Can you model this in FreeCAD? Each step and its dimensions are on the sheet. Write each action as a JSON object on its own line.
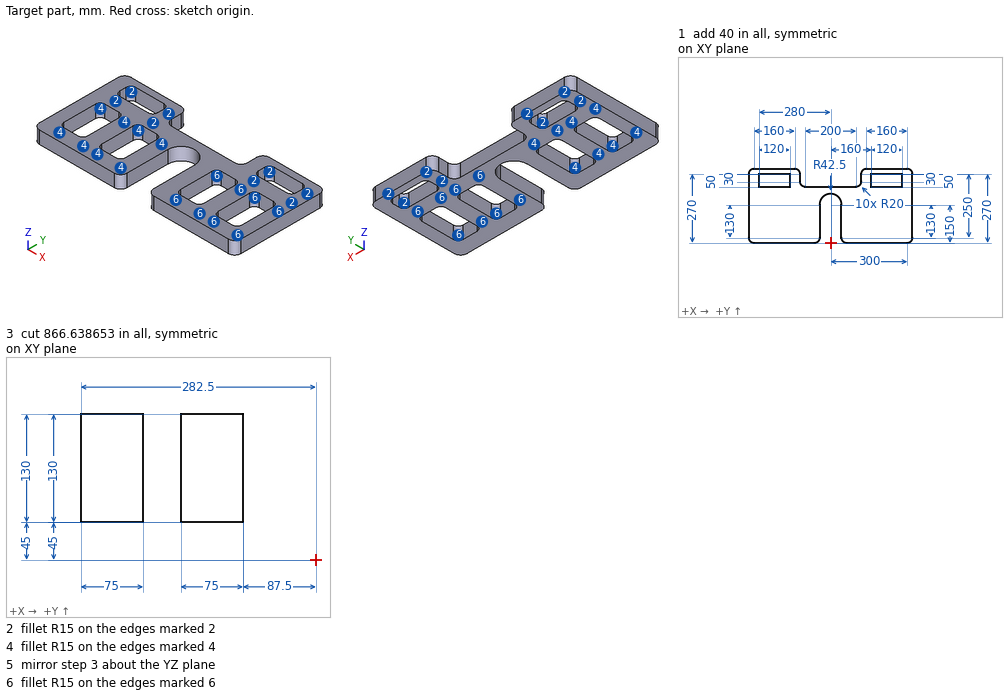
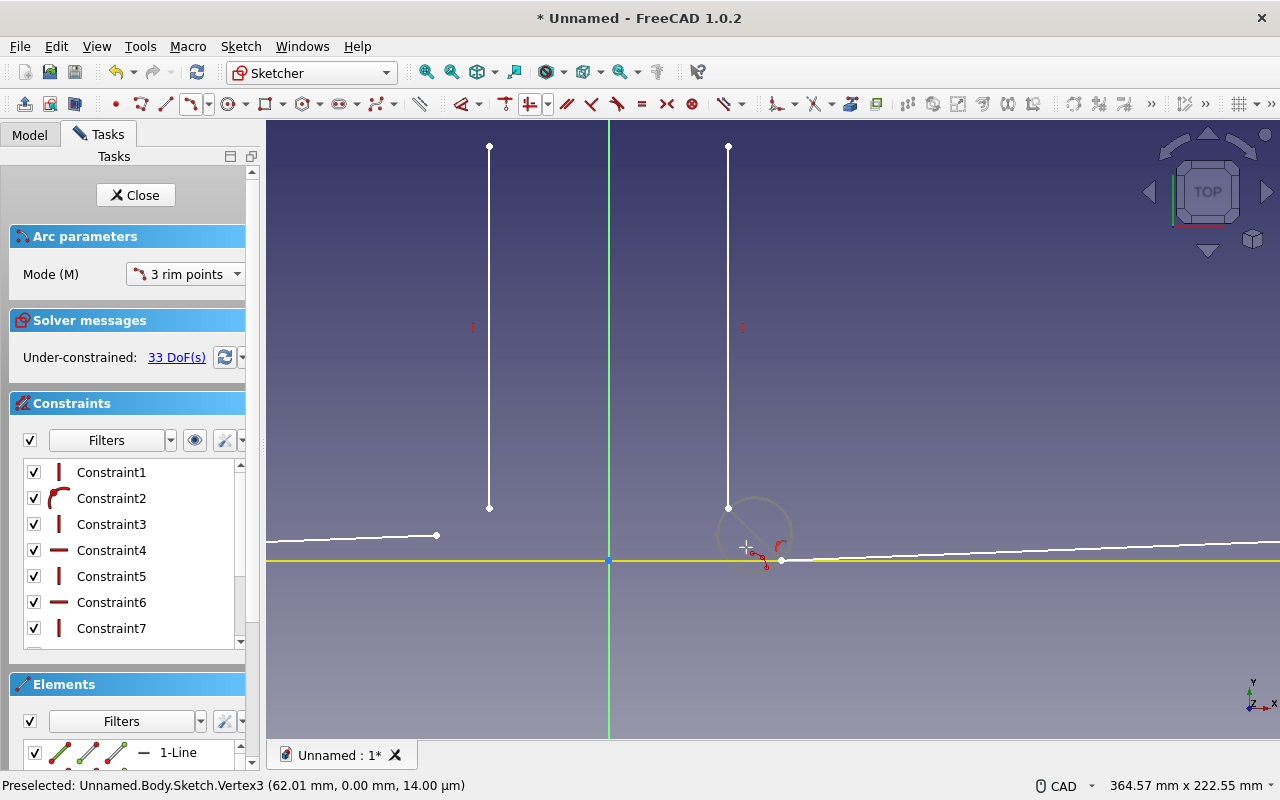
{"action": "left_click", "coordinate": [743, 544]}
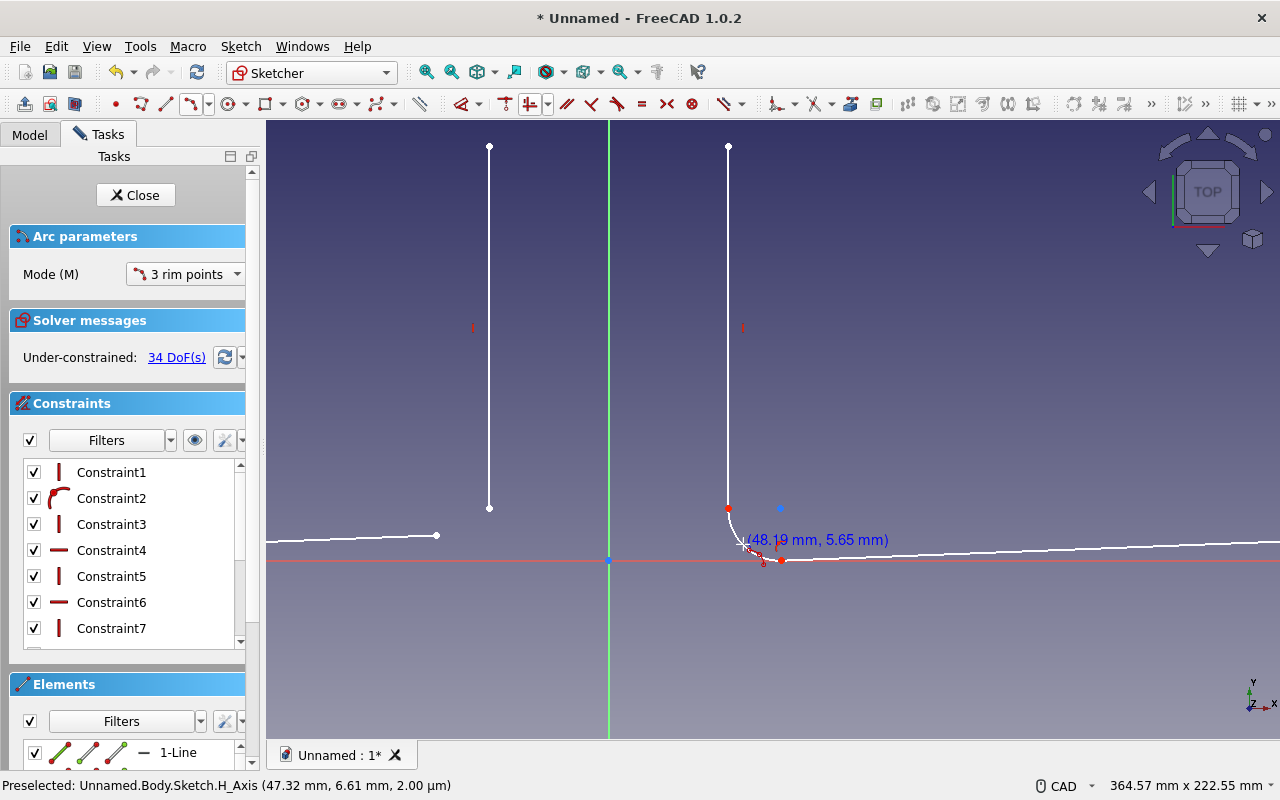
{"action": "scroll", "coordinate": [746, 547], "scroll_direction": "down", "scroll_amount": 6}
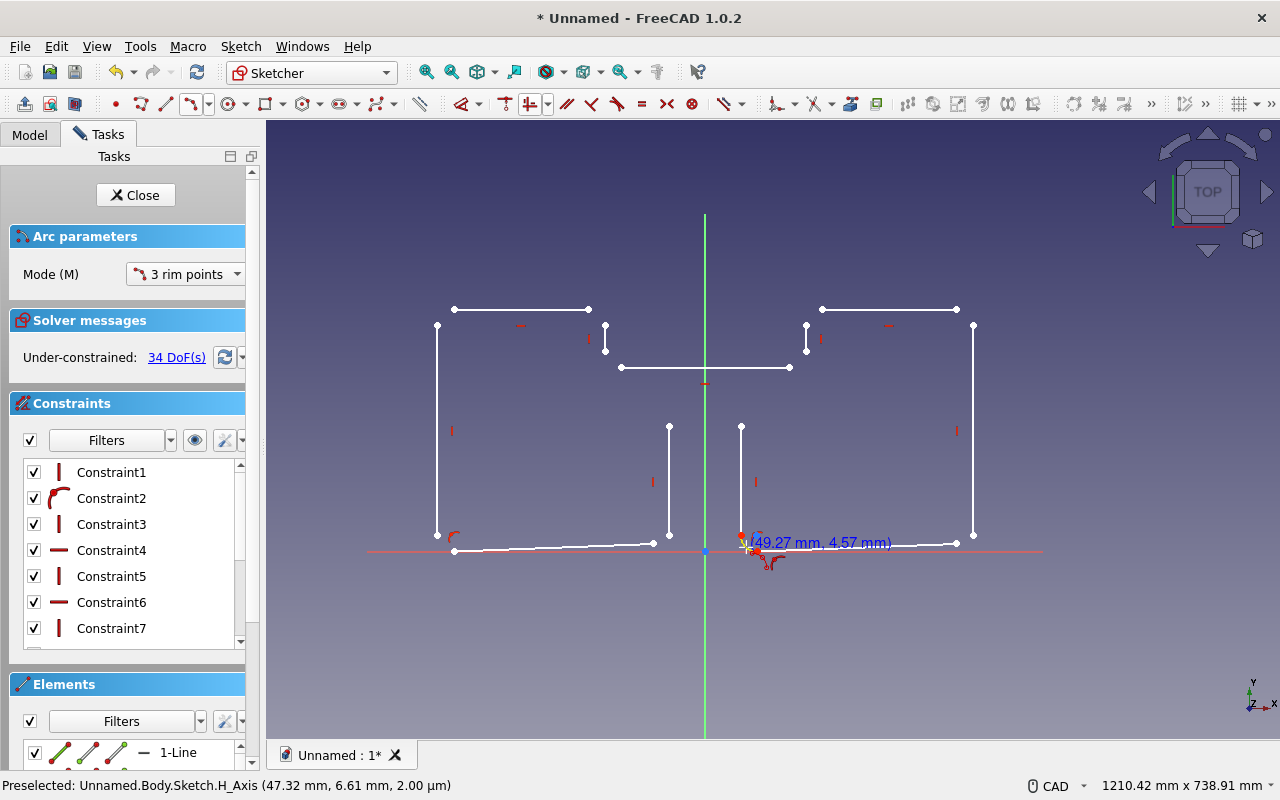
{"action": "left_click", "coordinate": [956, 544]}
{"action": "left_click", "coordinate": [973, 536]}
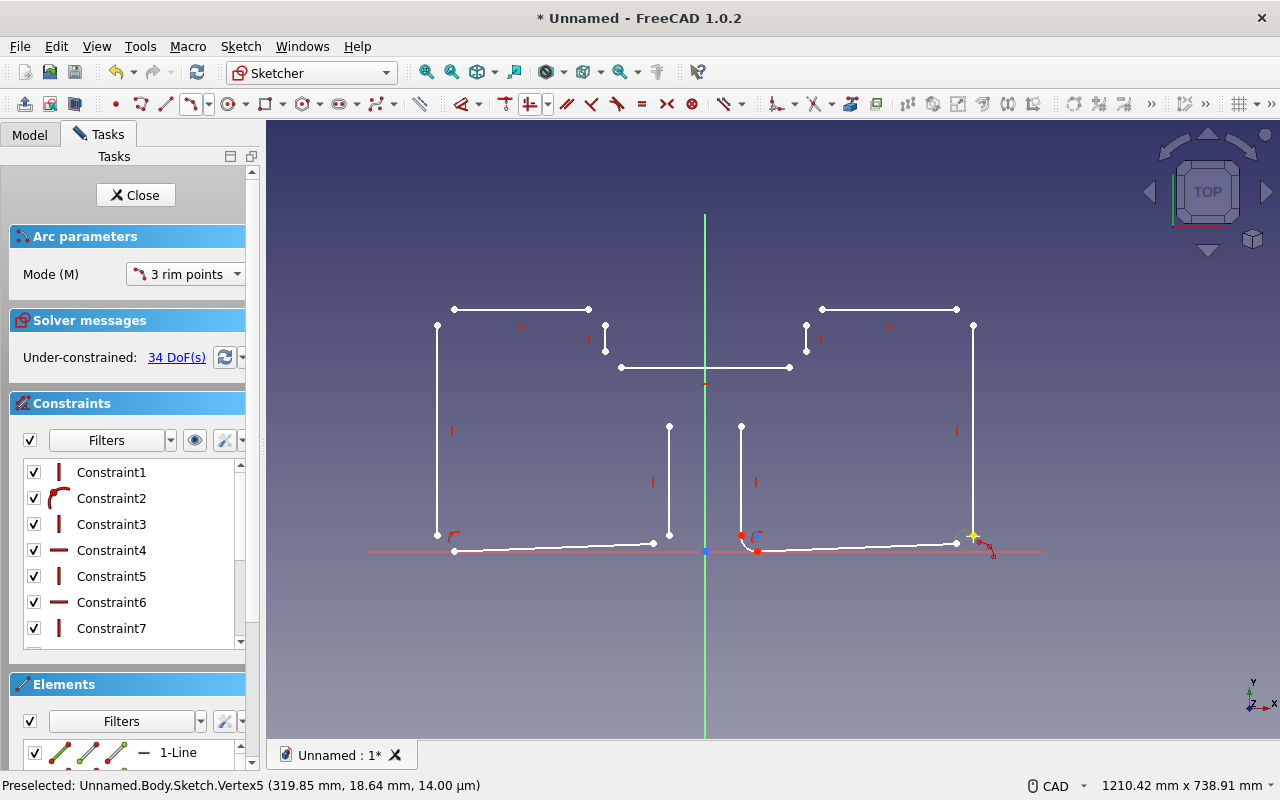
{"action": "scroll", "coordinate": [968, 547], "scroll_direction": "up", "scroll_amount": 6}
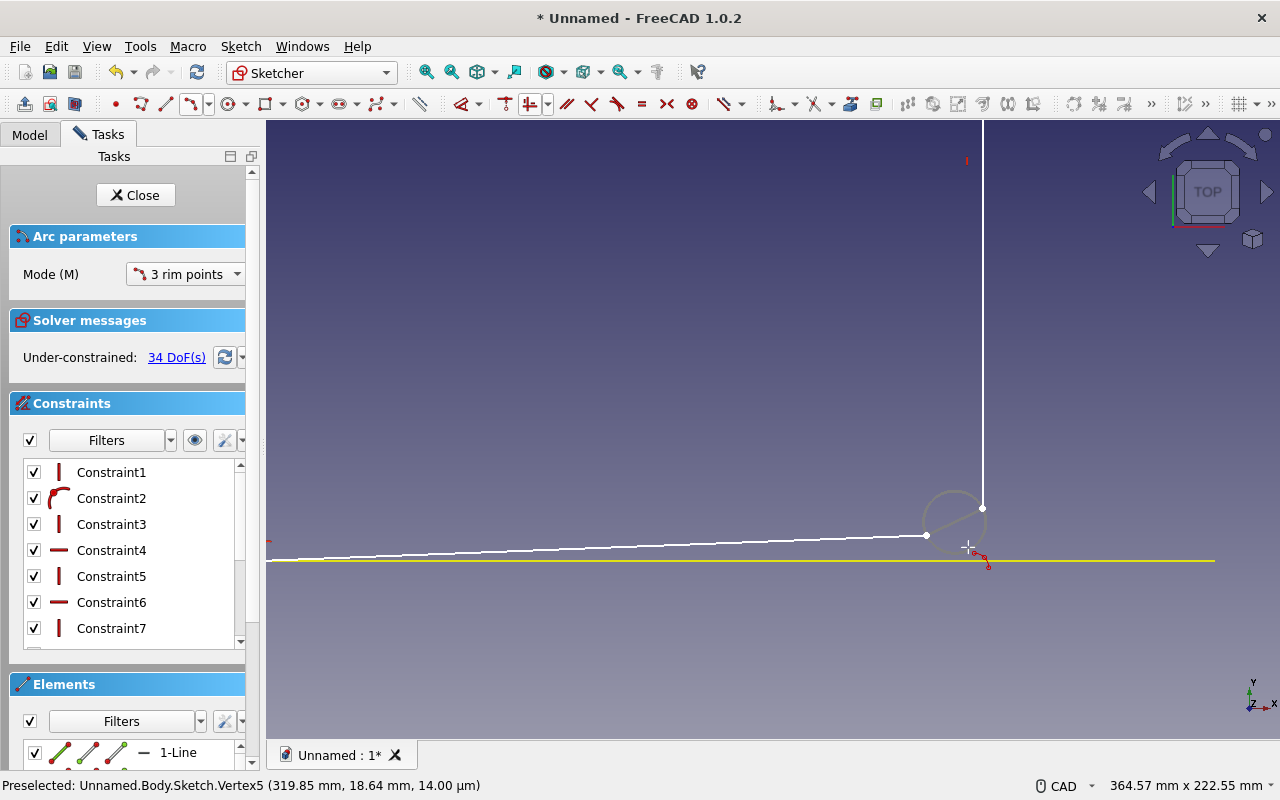
{"action": "left_click", "coordinate": [967, 544]}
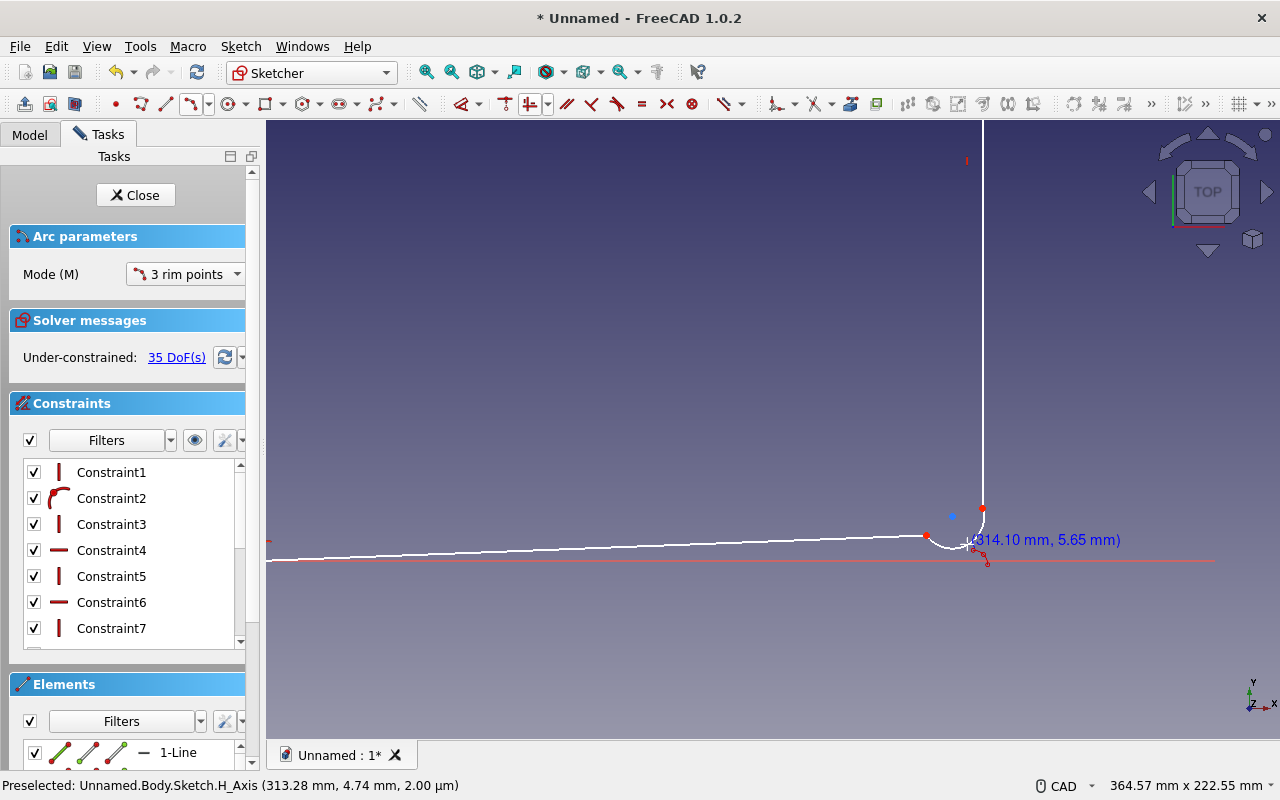
{"action": "scroll", "coordinate": [968, 547], "scroll_direction": "down", "scroll_amount": 6}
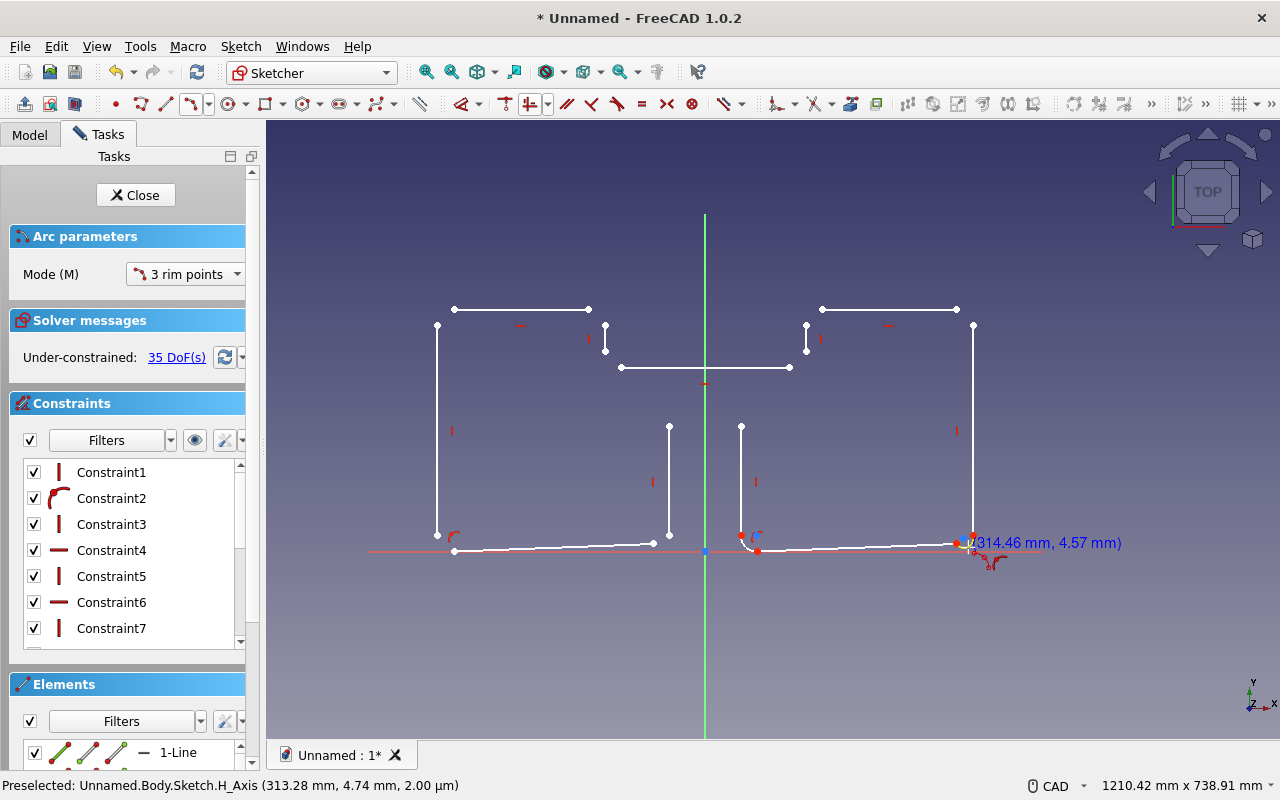
{"action": "left_click", "coordinate": [973, 326]}
{"action": "left_click", "coordinate": [956, 310]}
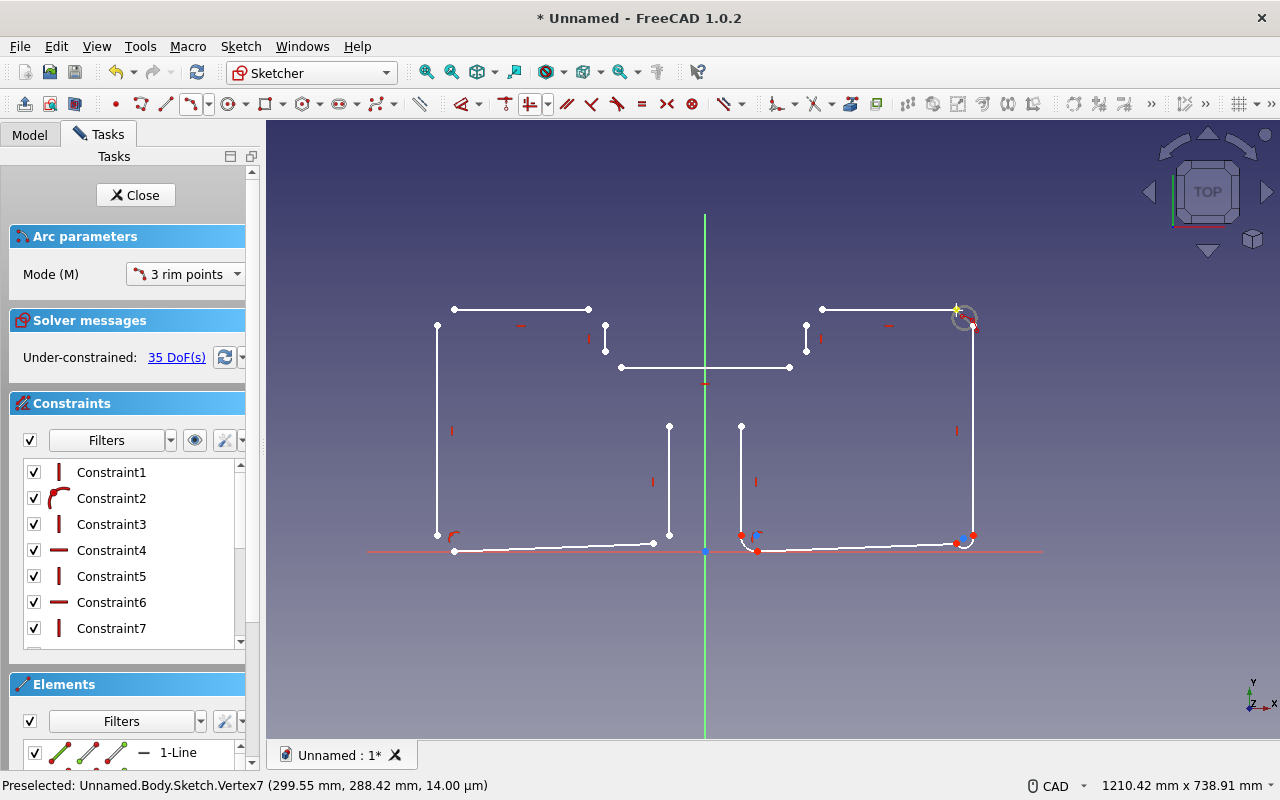
{"action": "scroll", "coordinate": [968, 314], "scroll_direction": "up", "scroll_amount": 6}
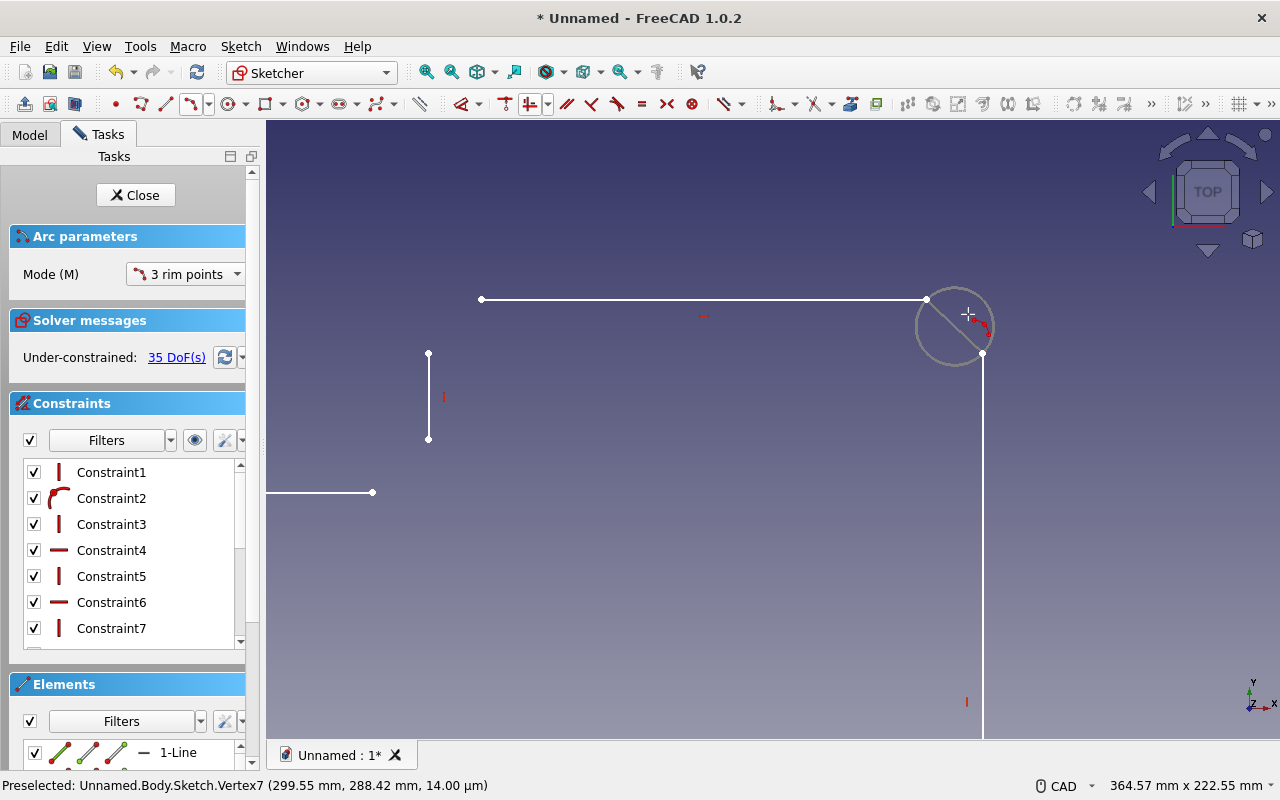
{"action": "left_click", "coordinate": [967, 312]}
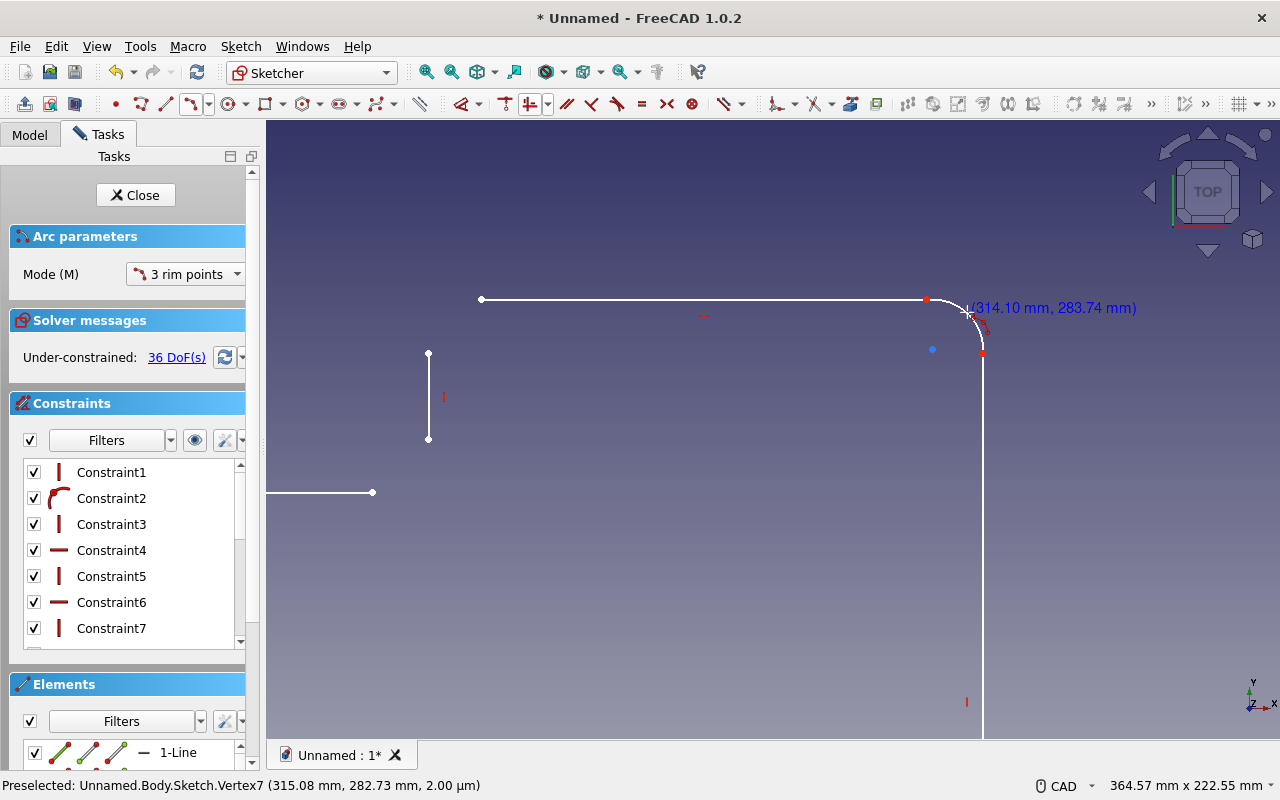
{"action": "left_click", "coordinate": [482, 300]}
{"action": "left_click", "coordinate": [429, 353]}
{"action": "left_click", "coordinate": [443, 312]}